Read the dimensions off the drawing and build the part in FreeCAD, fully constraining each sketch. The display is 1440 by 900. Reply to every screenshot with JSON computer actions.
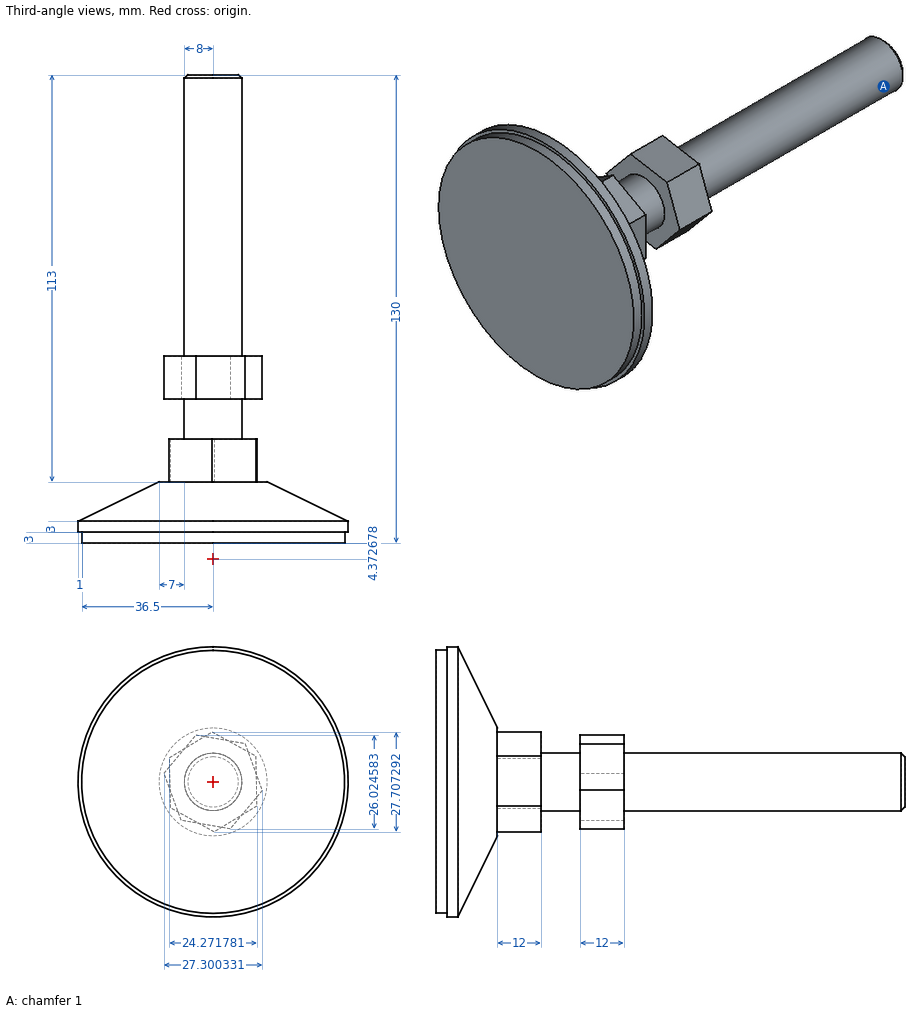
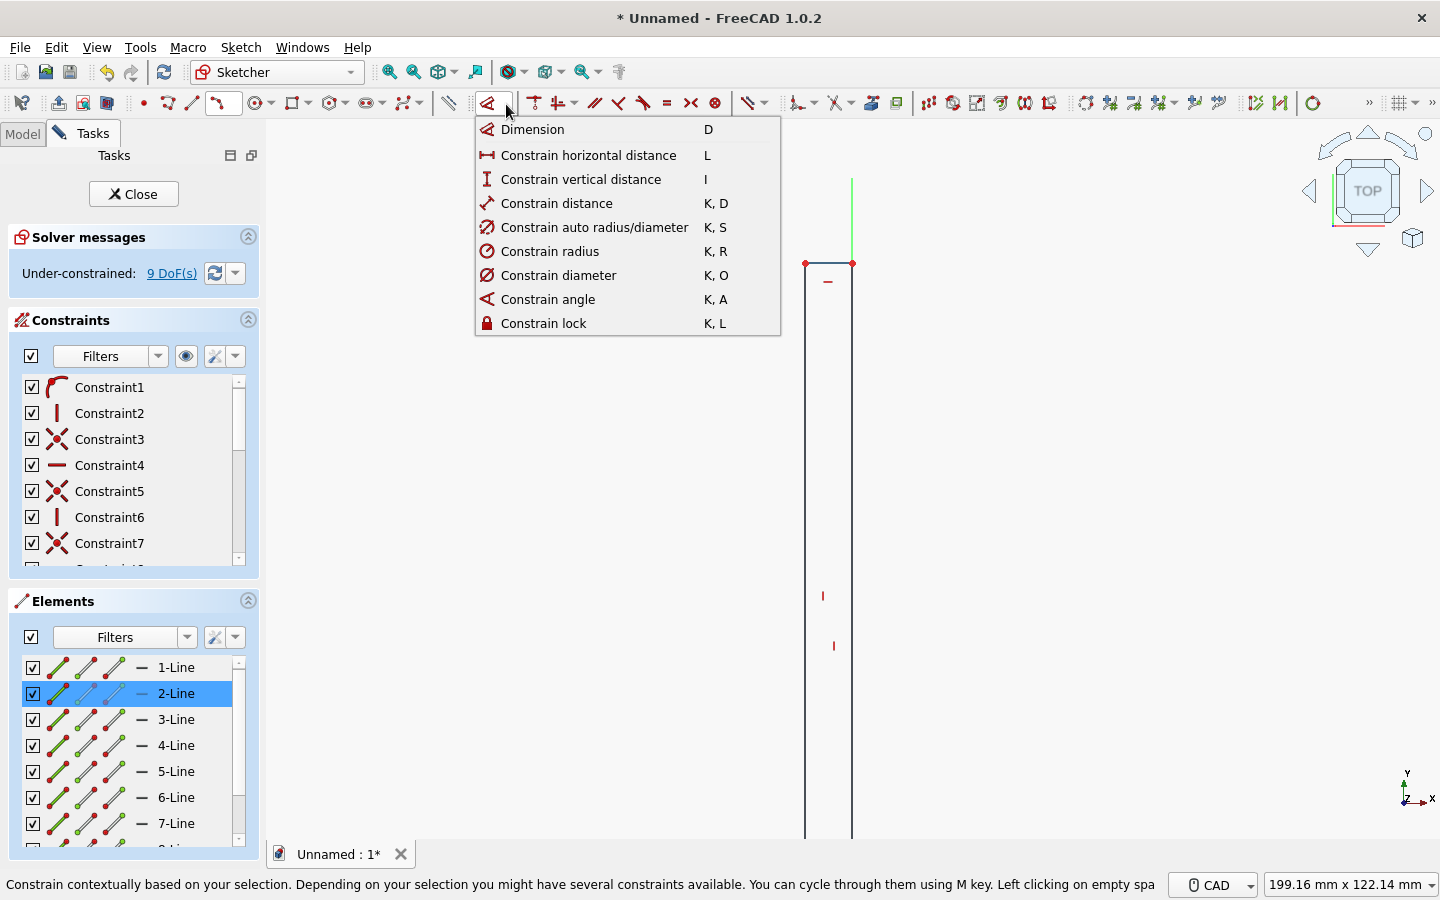
{"action": "left_click", "coordinate": [628, 155]}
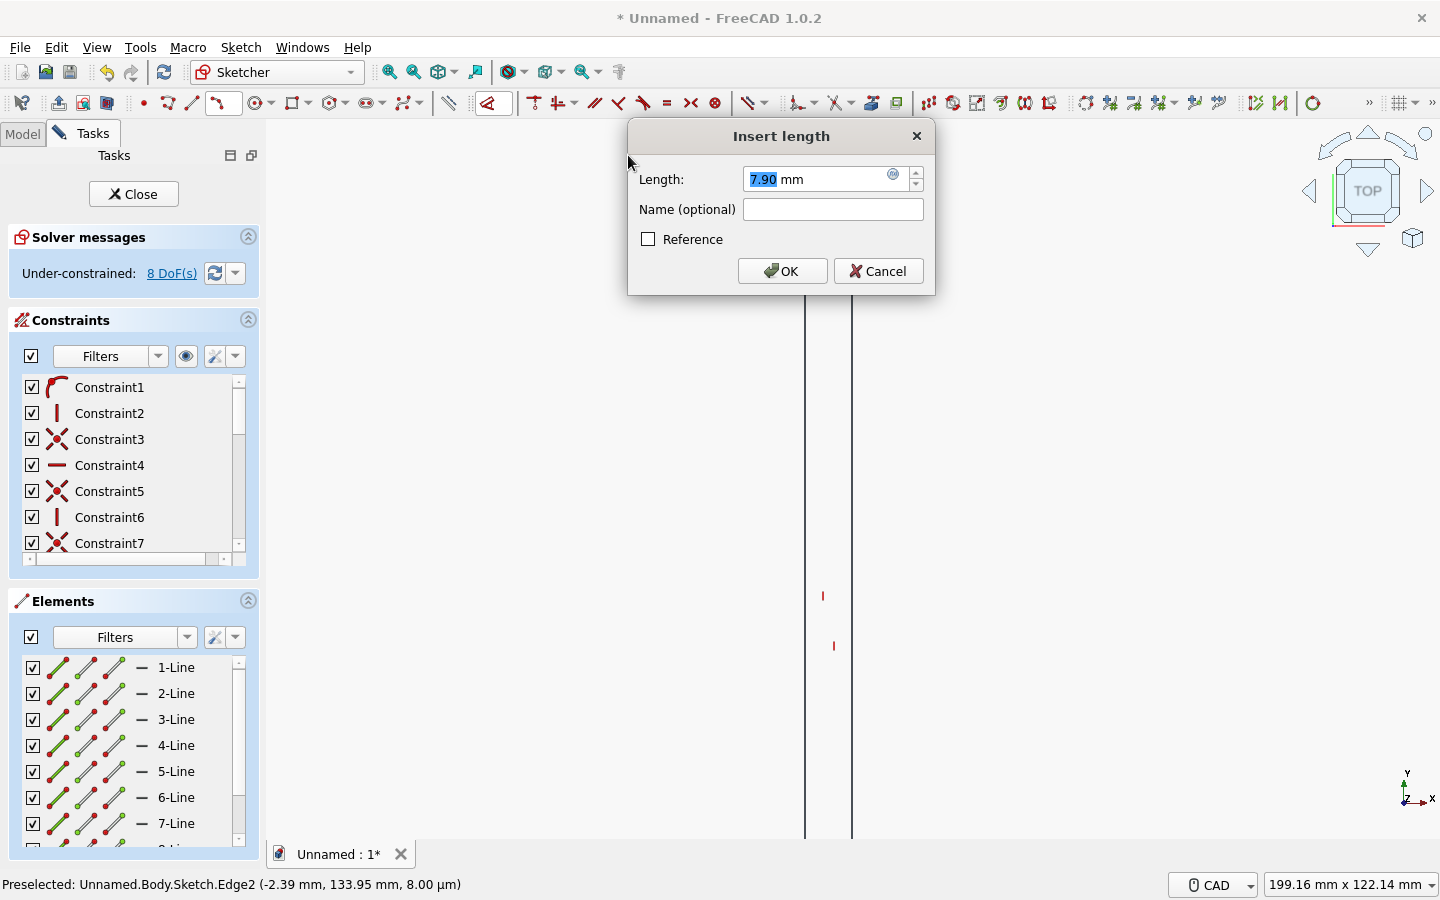
{"action": "type", "text": "8"}
{"action": "key", "text": "Return"}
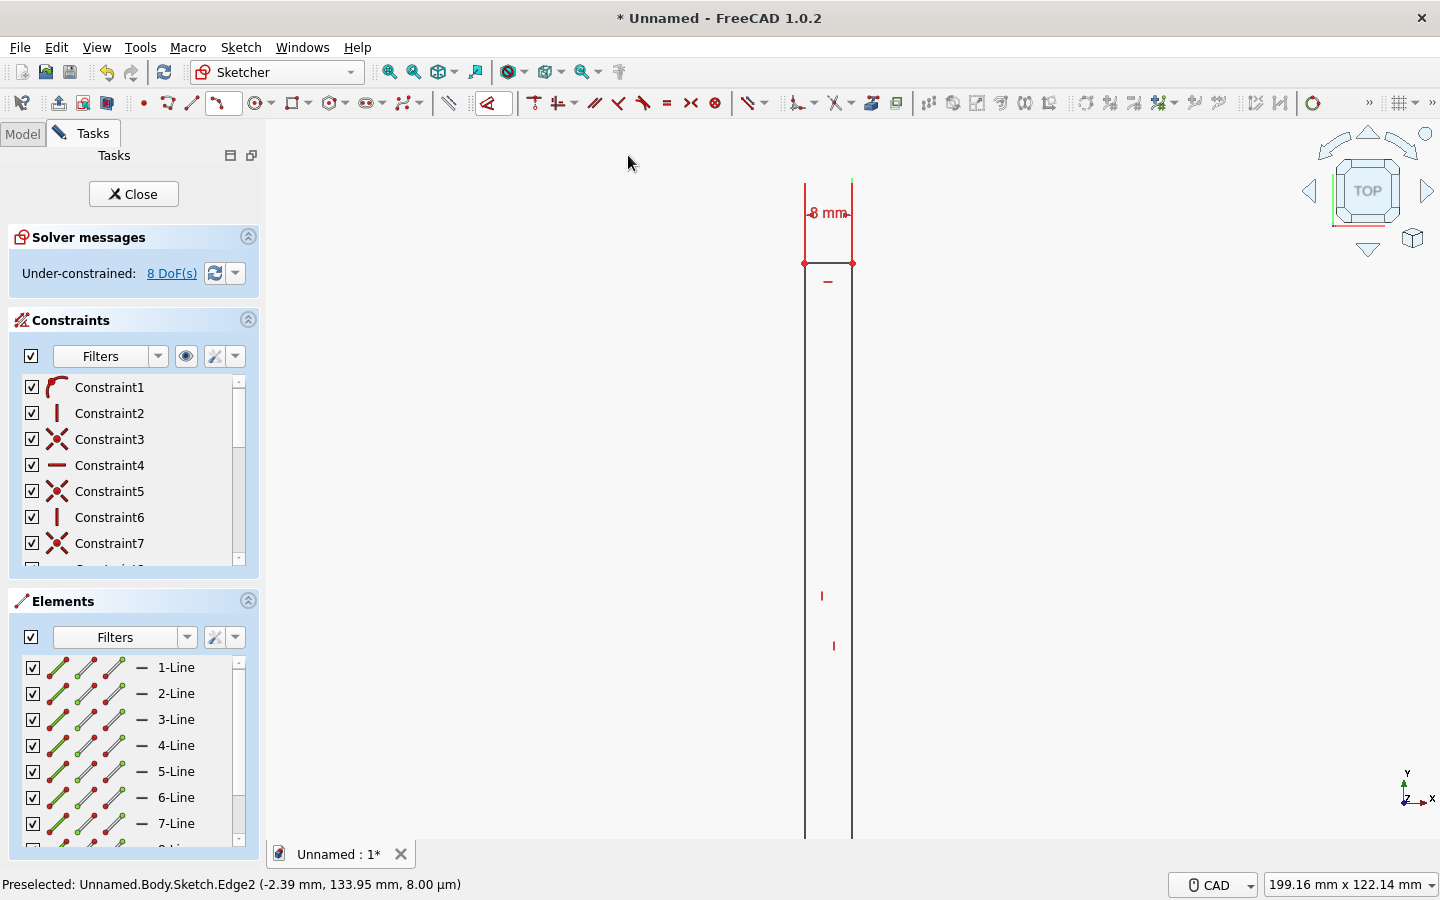
{"action": "scroll", "coordinate": [837, 263], "scroll_direction": "down", "scroll_amount": 3}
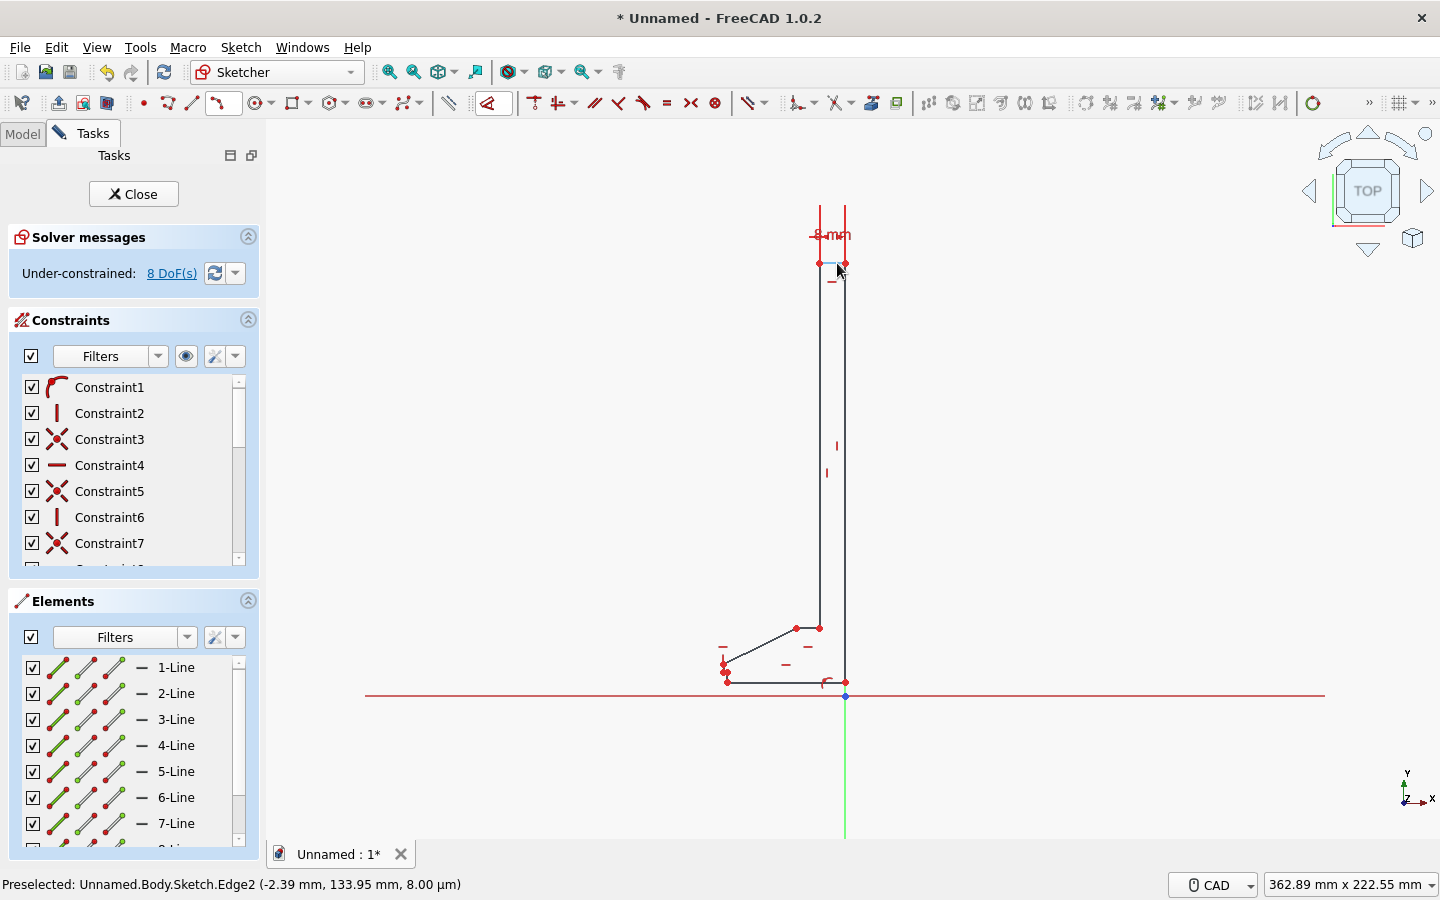
{"action": "scroll", "coordinate": [813, 628], "scroll_direction": "up", "scroll_amount": 4}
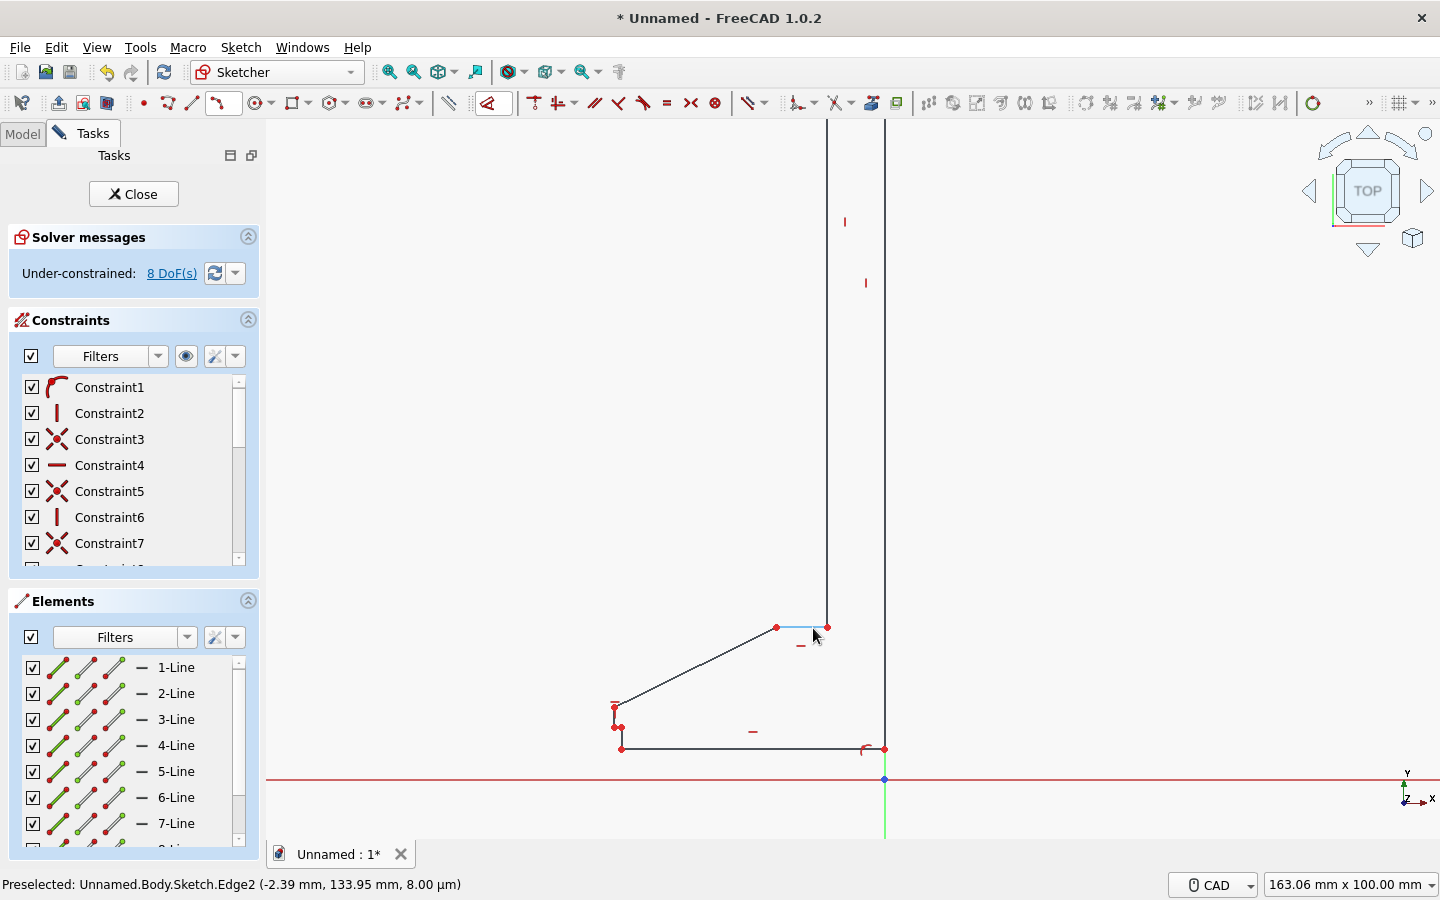
{"action": "left_click", "coordinate": [812, 627]}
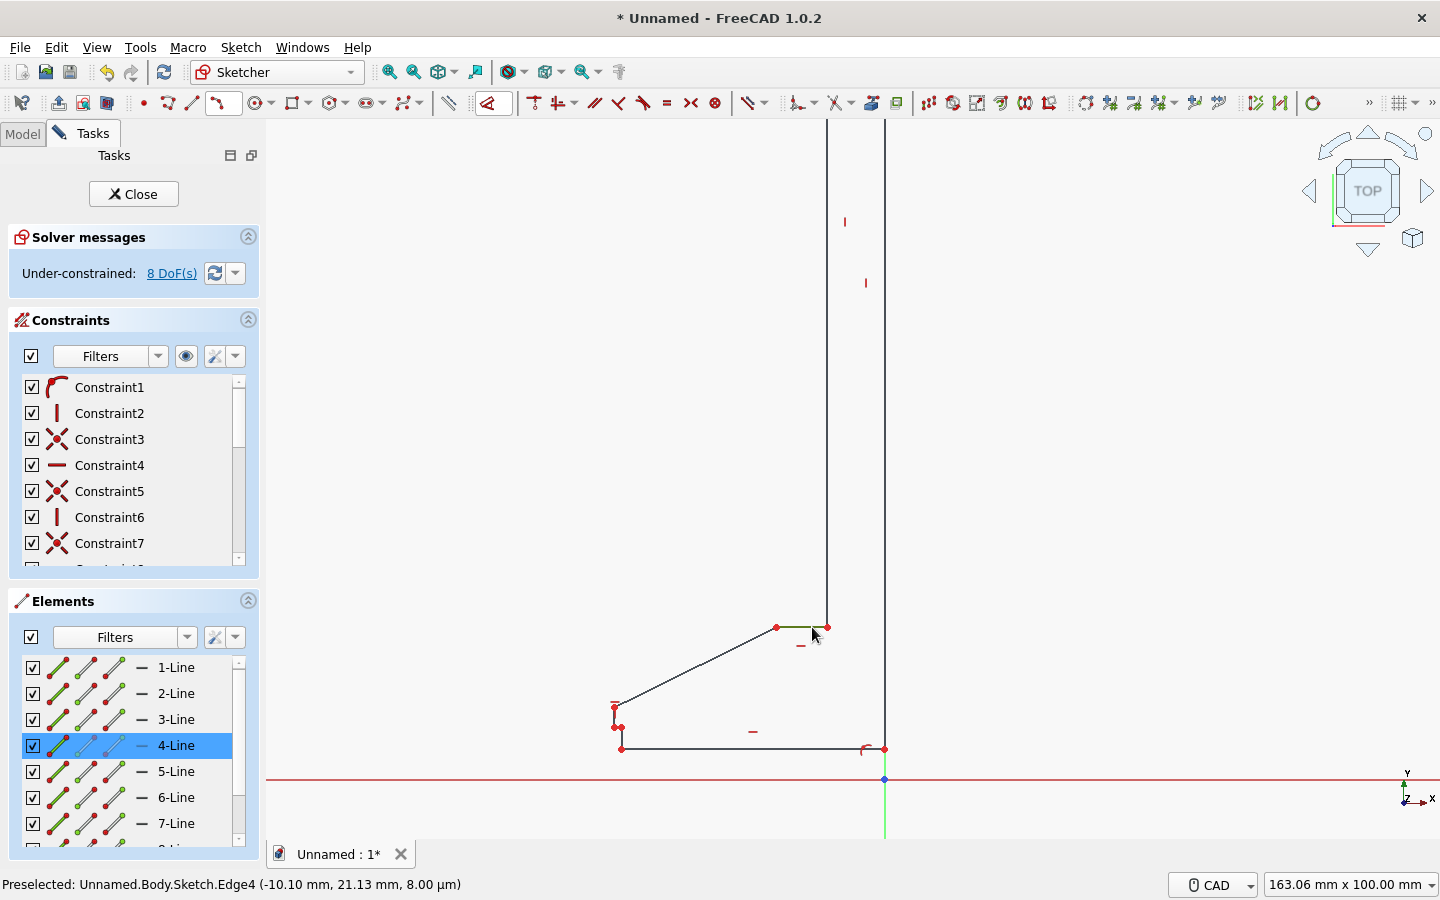
{"action": "left_click", "coordinate": [506, 104]}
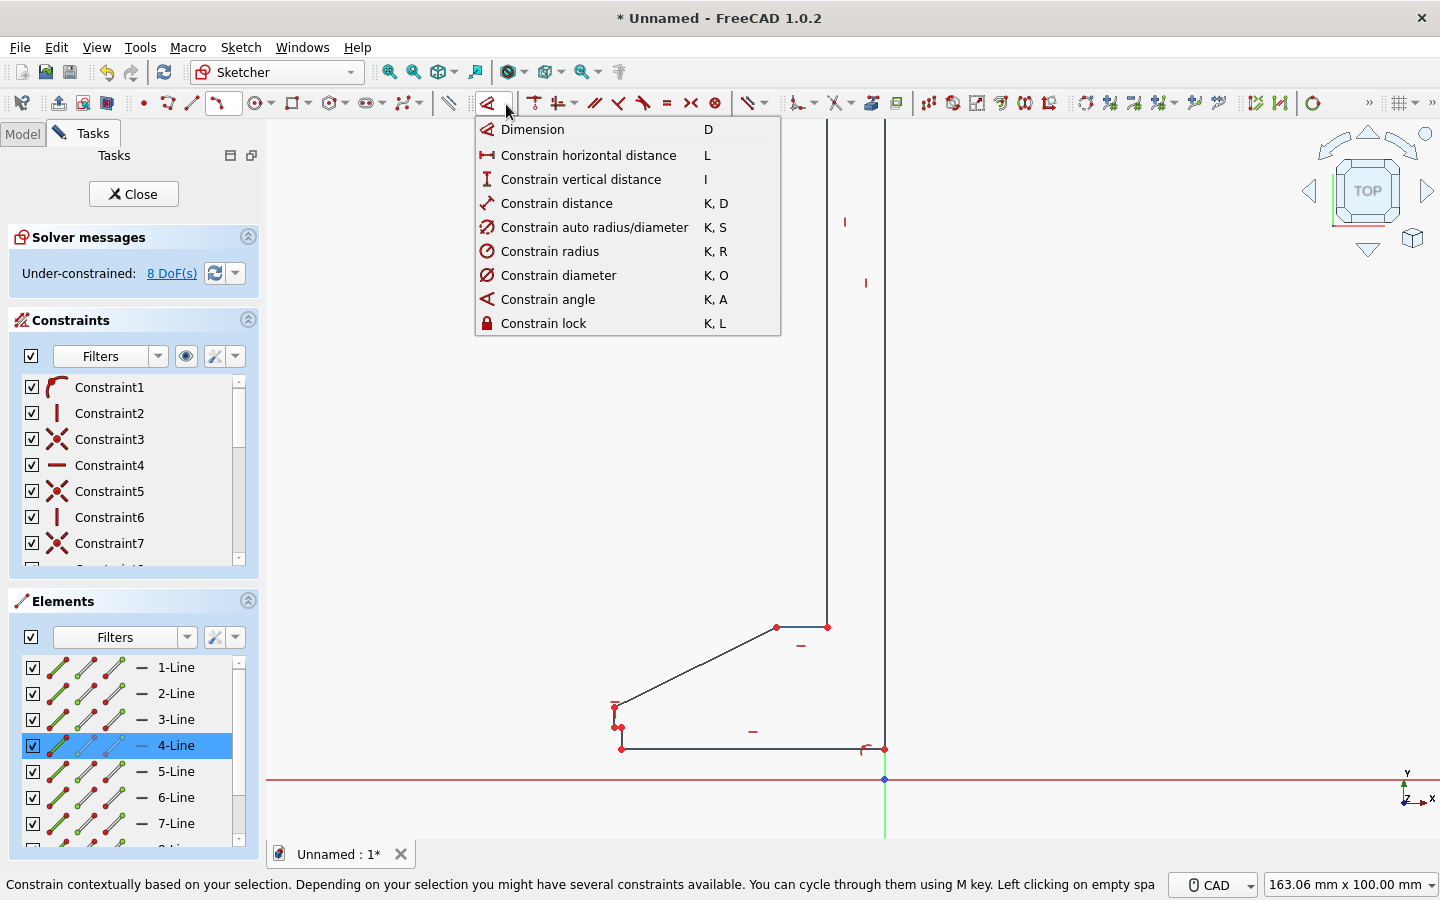
{"action": "left_click", "coordinate": [628, 155]}